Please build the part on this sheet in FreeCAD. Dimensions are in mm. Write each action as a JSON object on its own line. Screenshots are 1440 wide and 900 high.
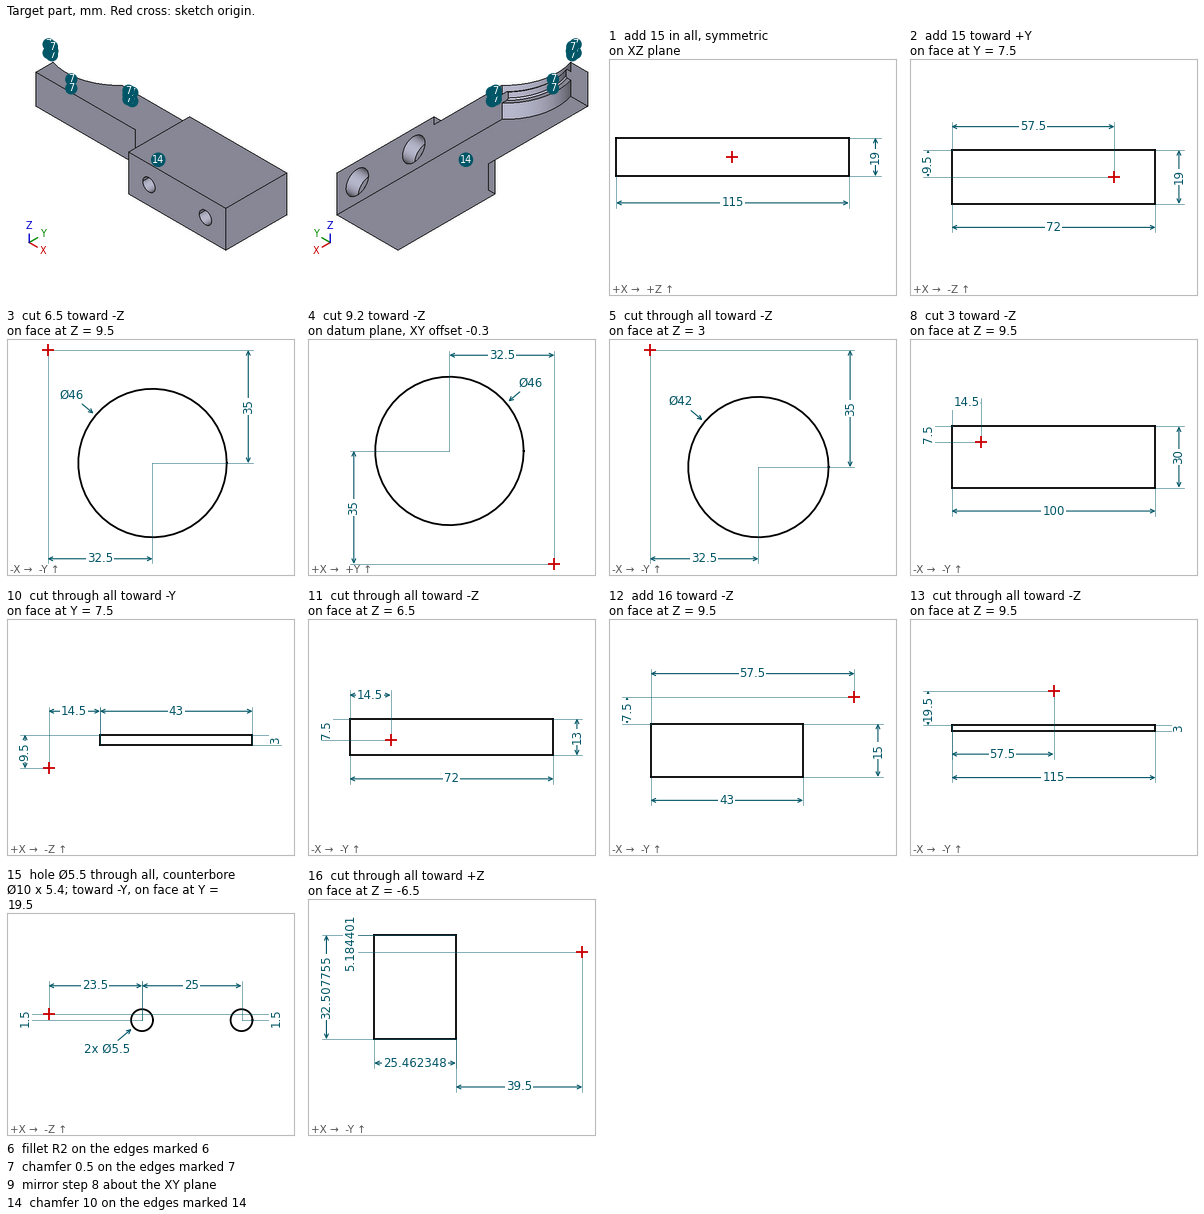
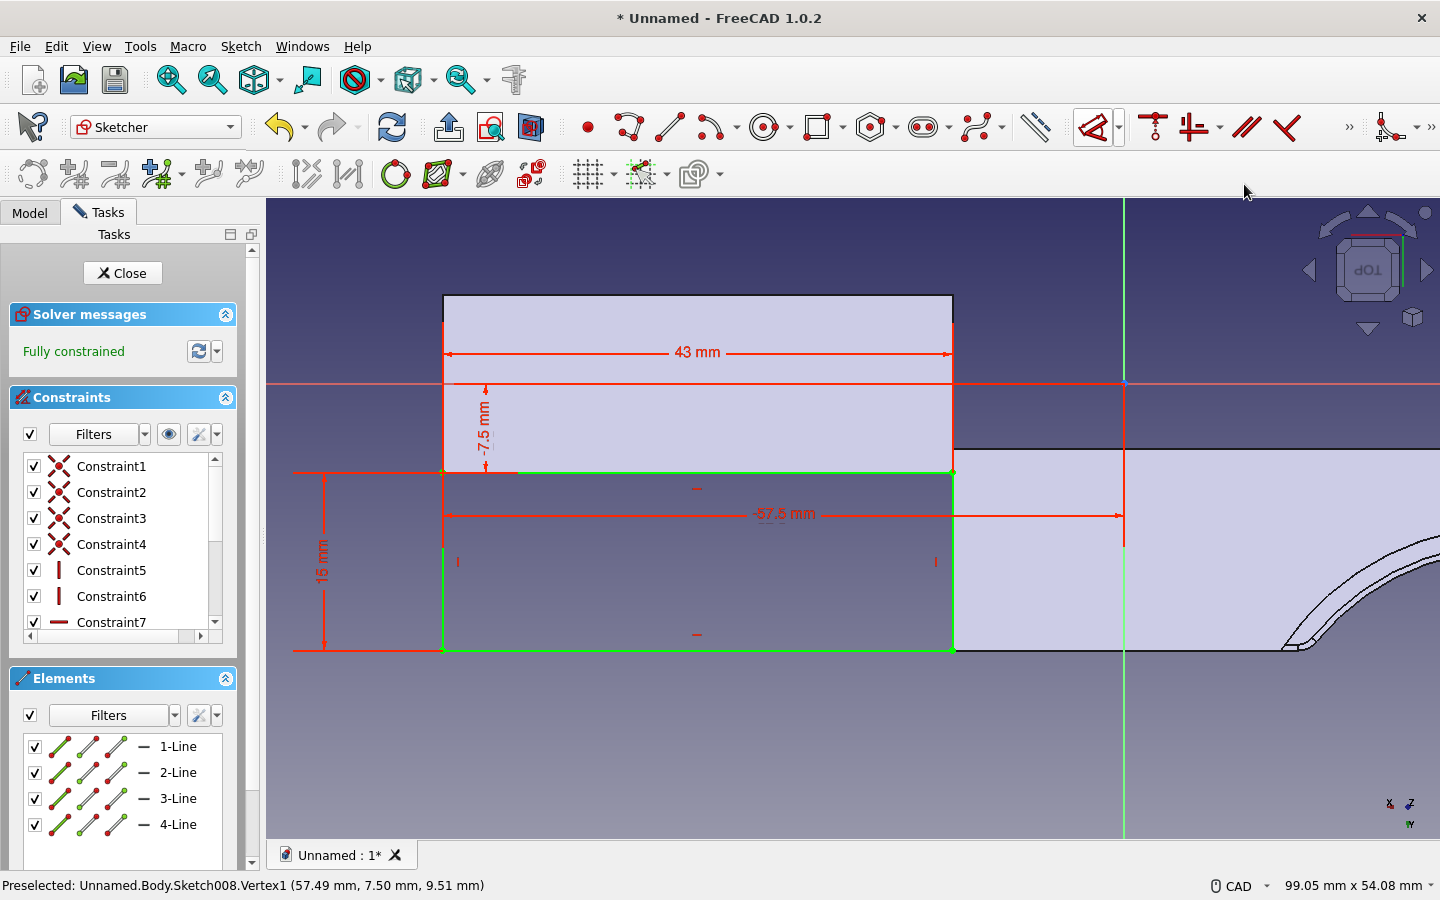
{"action": "left_click", "coordinate": [123, 273]}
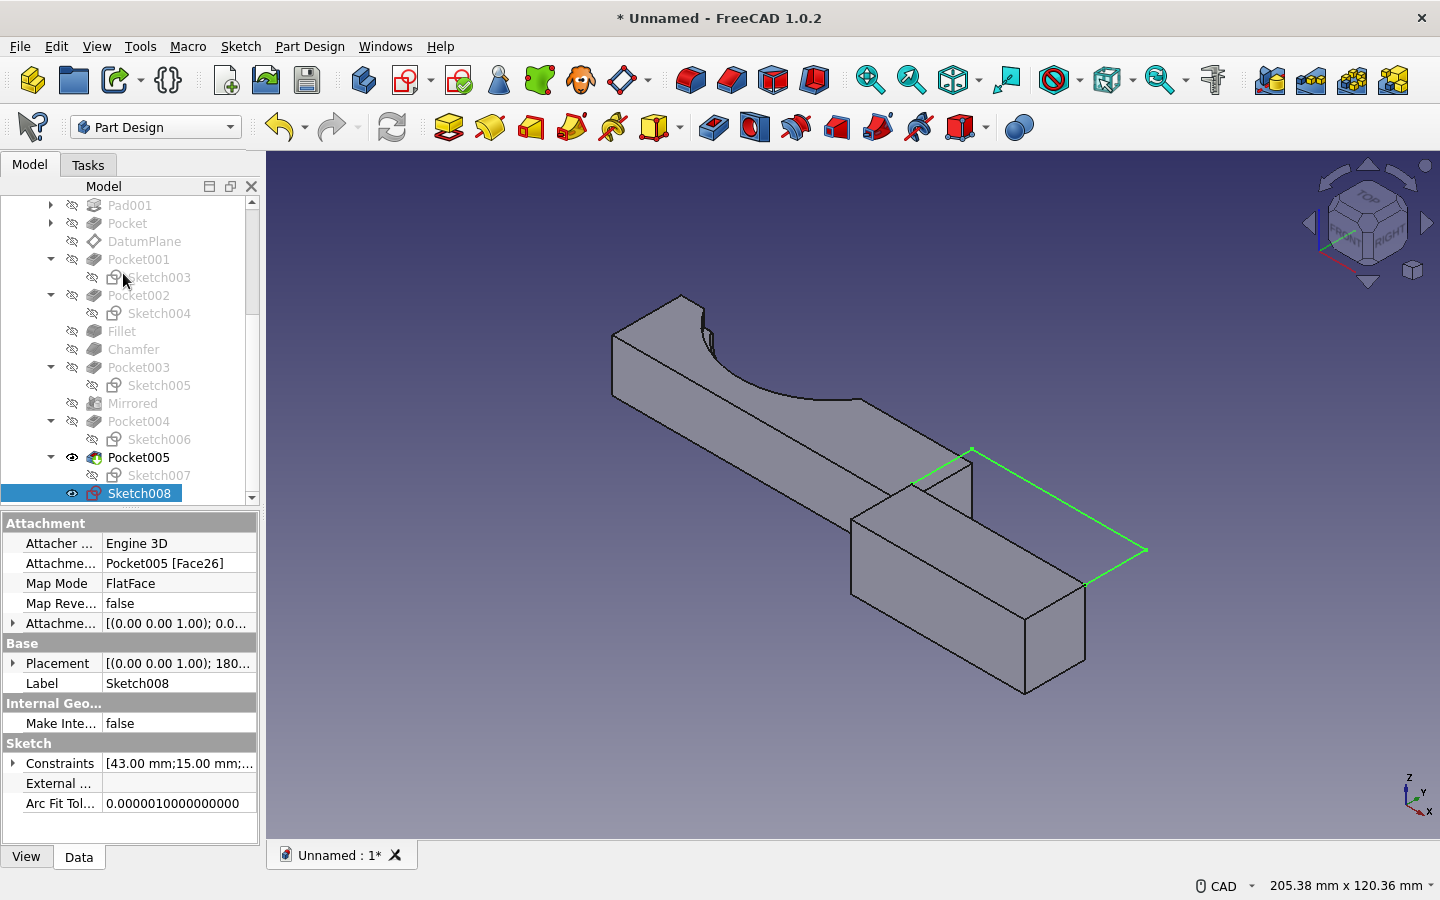
{"action": "left_click", "coordinate": [449, 128]}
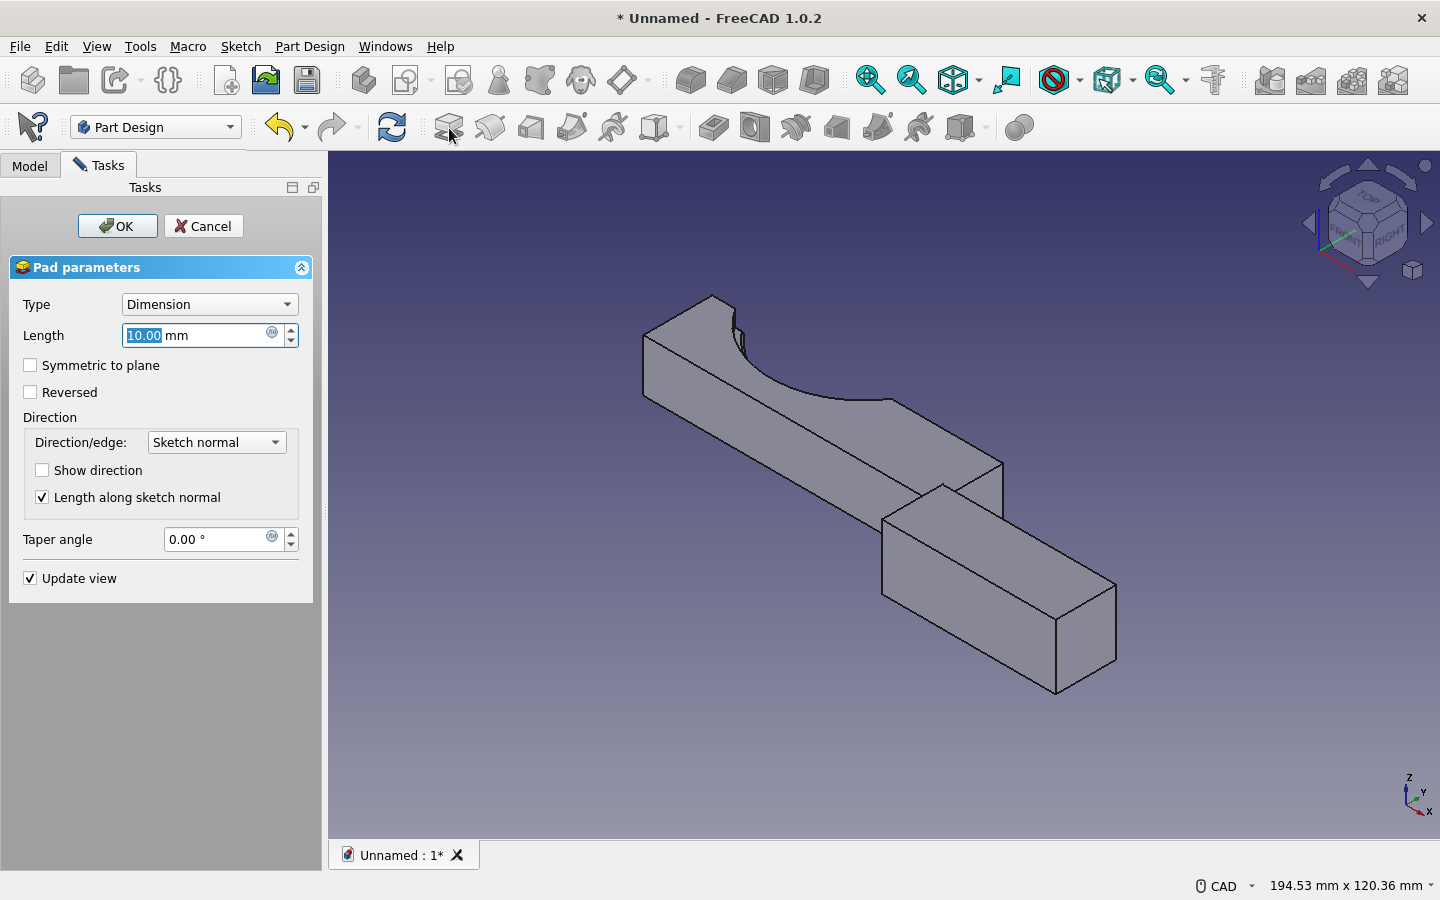
{"action": "type", "text": "16"}
{"action": "key", "text": "Tab"}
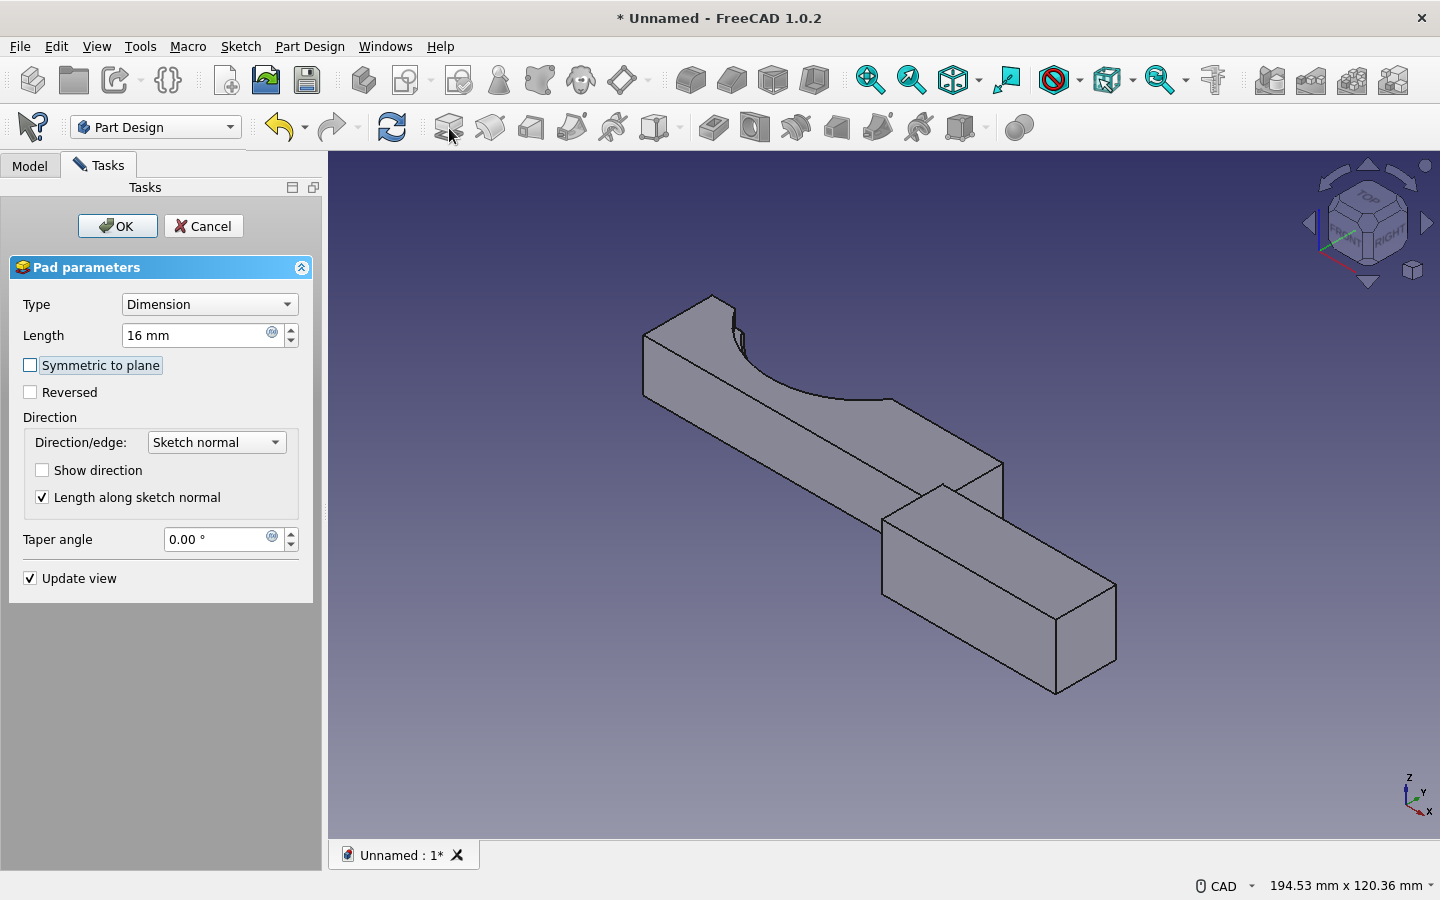
{"action": "left_click", "coordinate": [31, 392]}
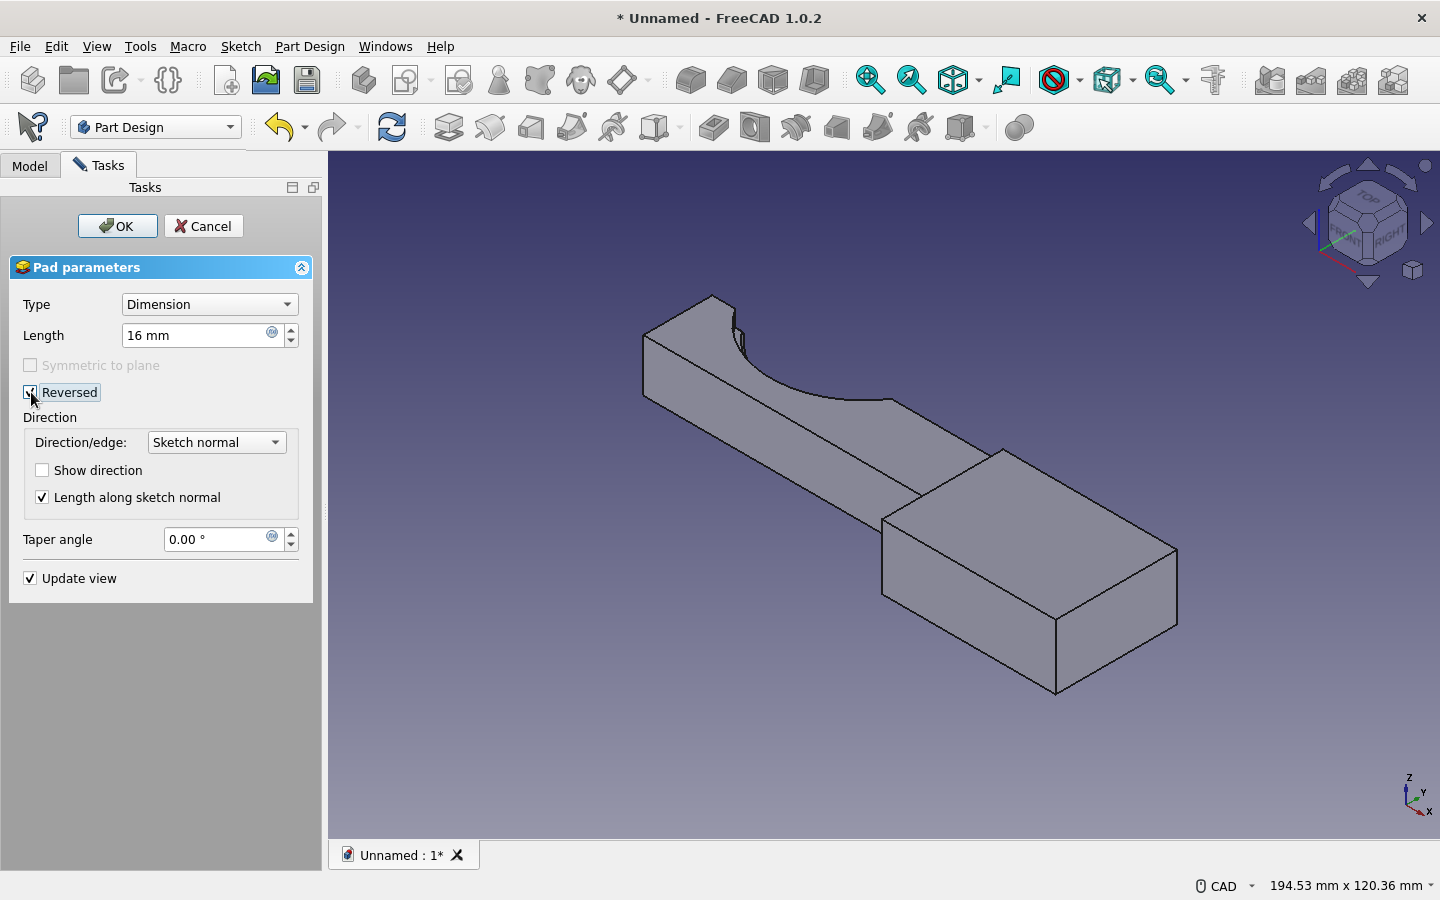
{"action": "left_click", "coordinate": [118, 226]}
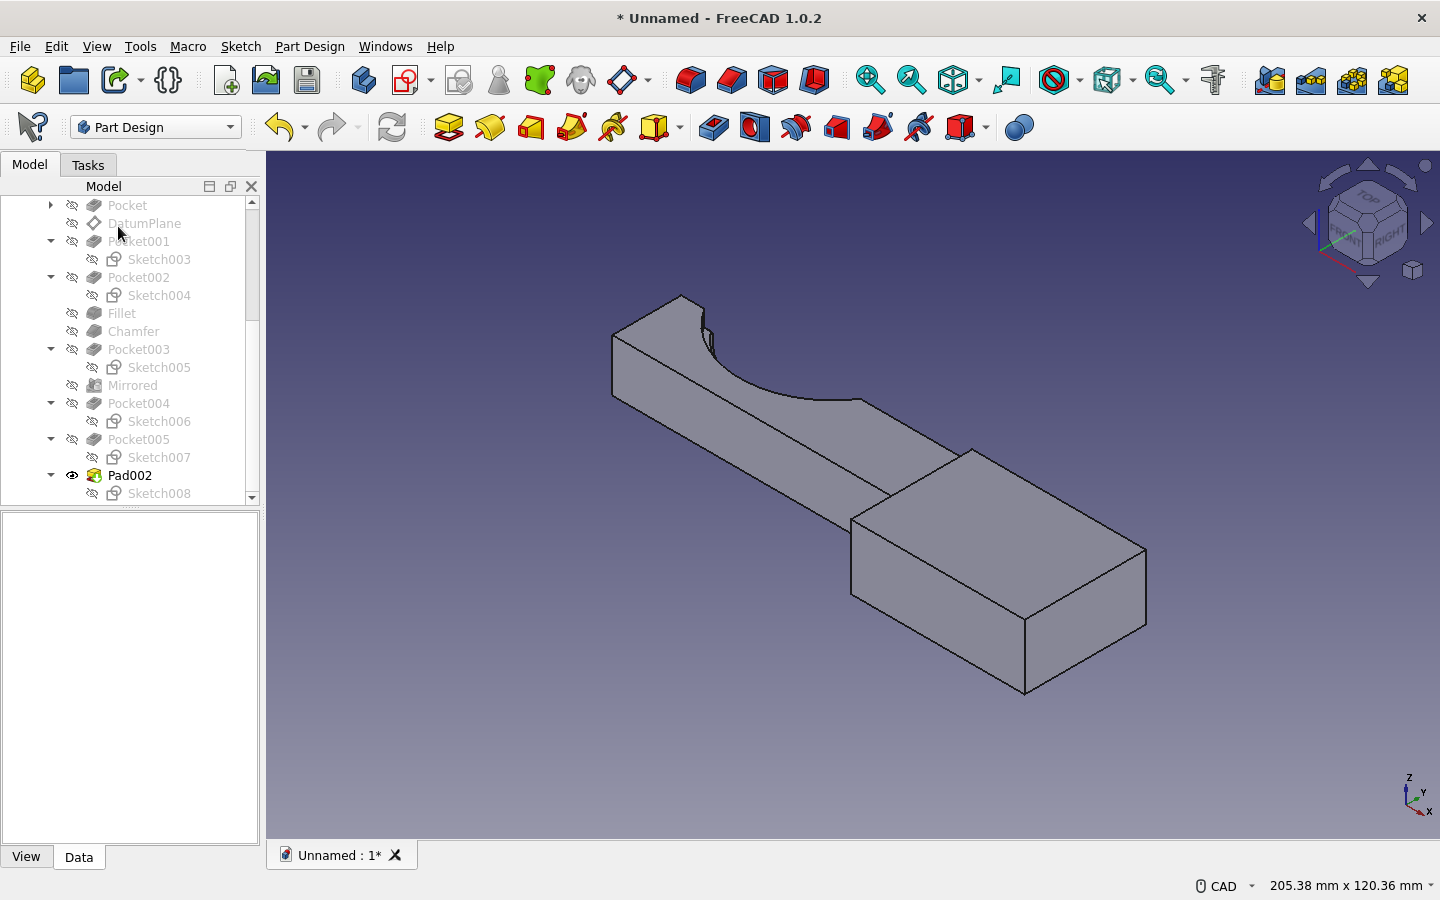
{"action": "left_click", "coordinate": [1023, 548]}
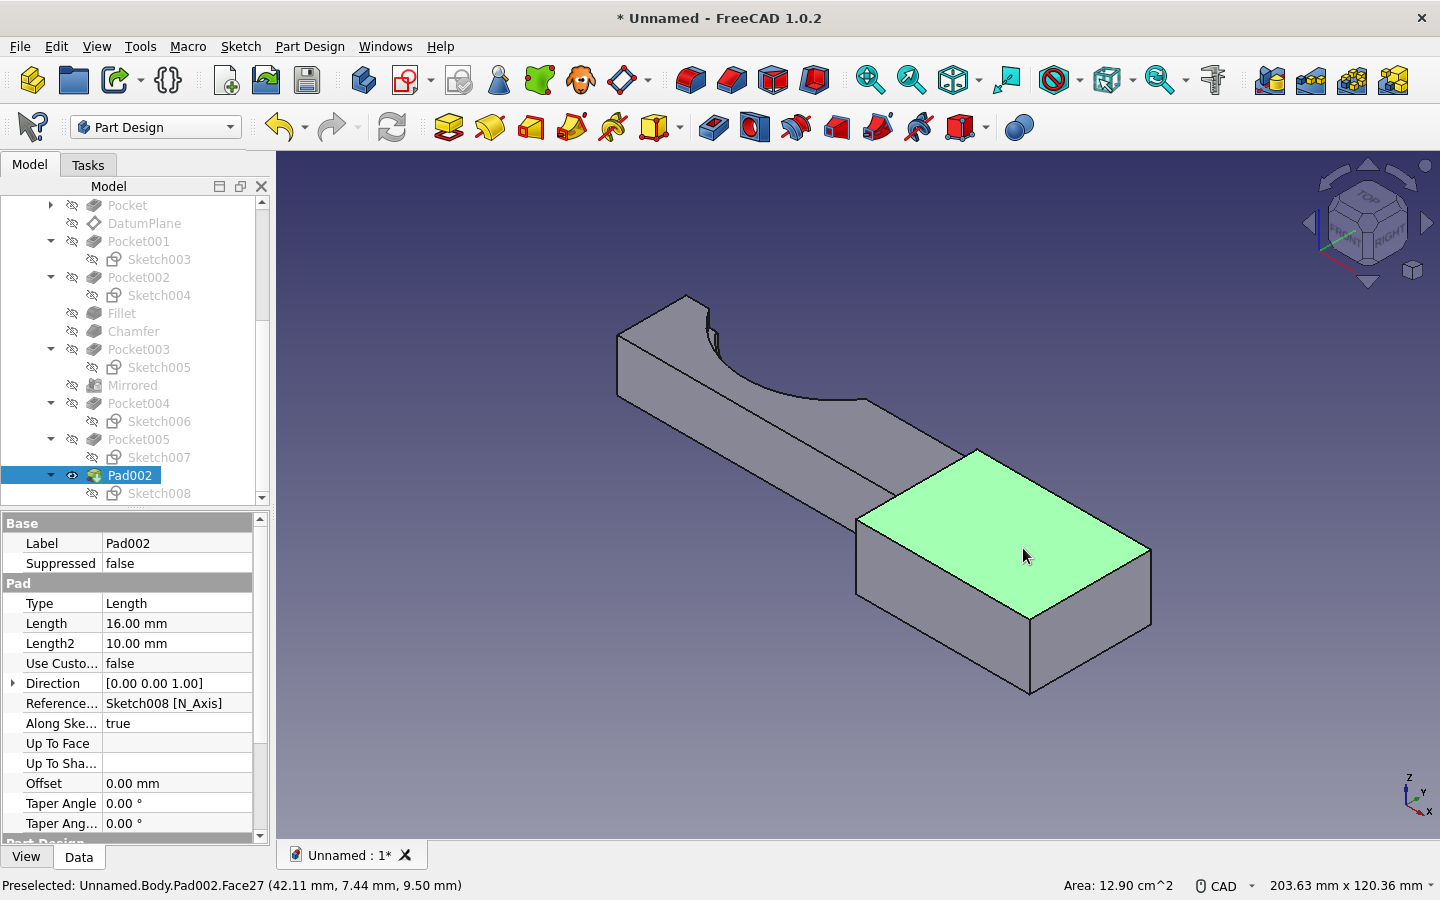
{"action": "left_click", "coordinate": [404, 80]}